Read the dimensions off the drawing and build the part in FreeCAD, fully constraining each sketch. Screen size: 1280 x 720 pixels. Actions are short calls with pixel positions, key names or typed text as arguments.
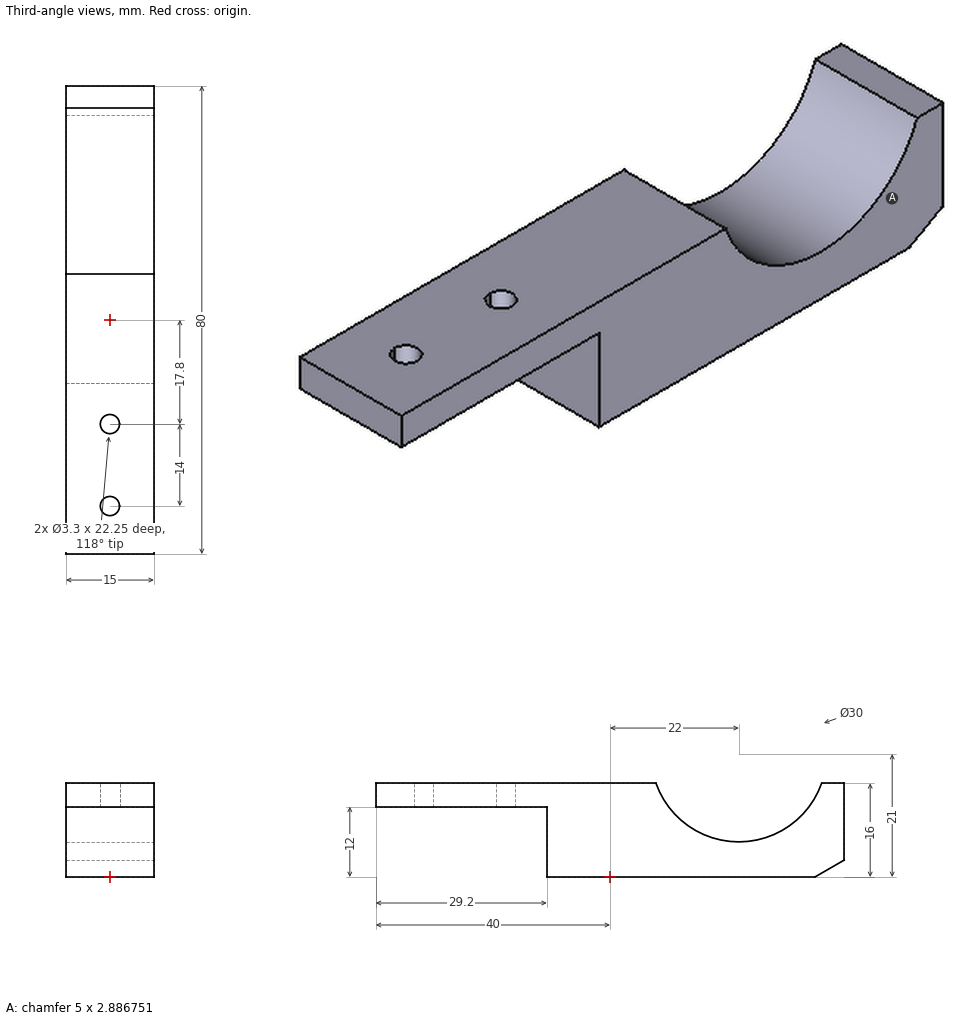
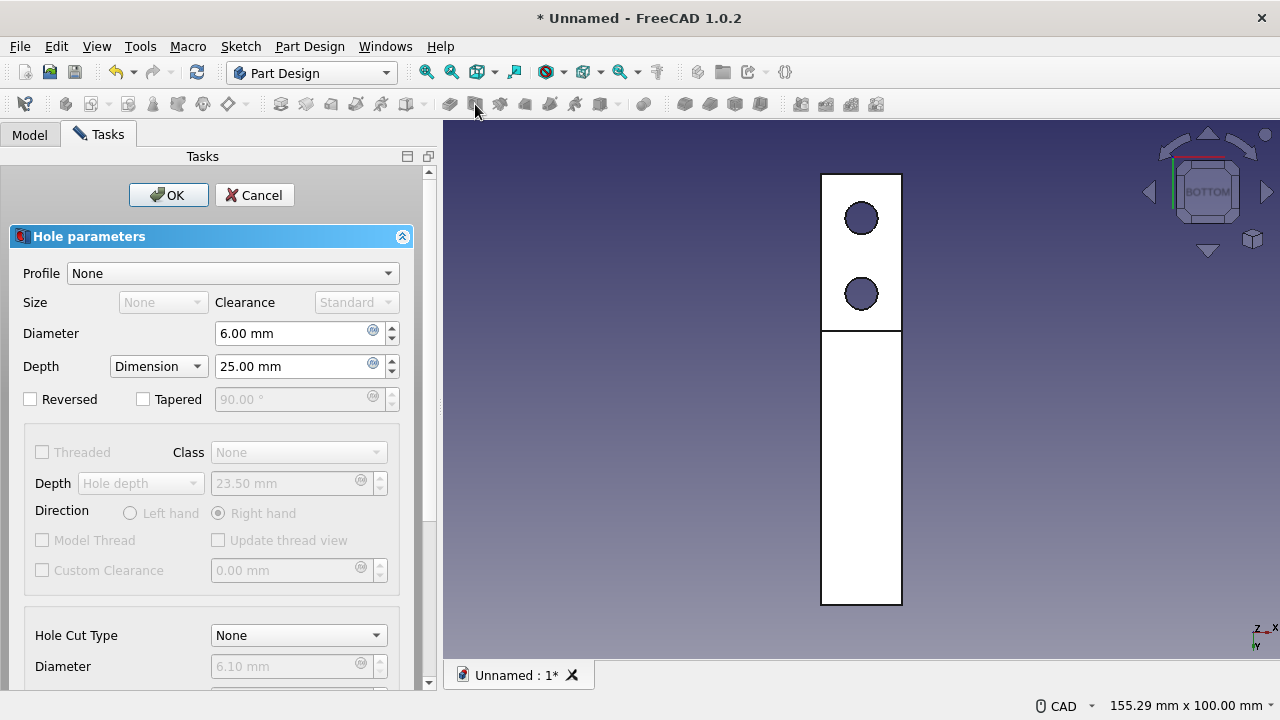
triple_click(300, 334)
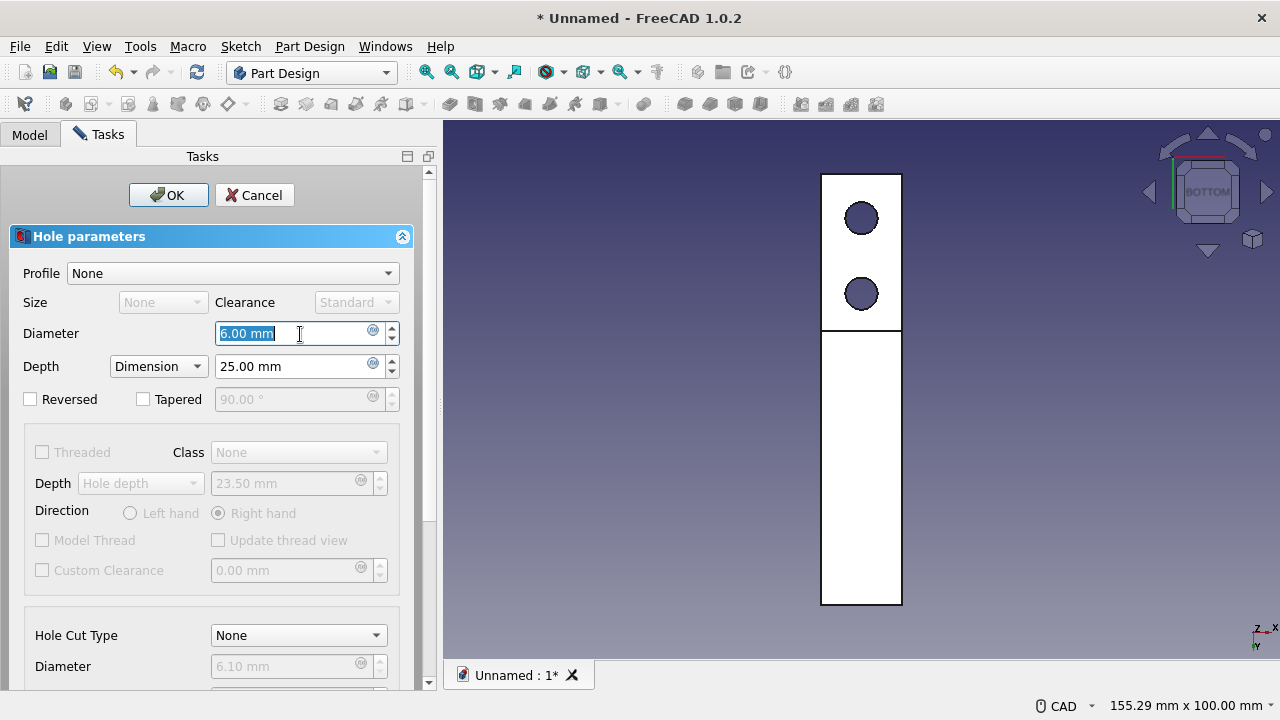
text(3.3)
key(Tab)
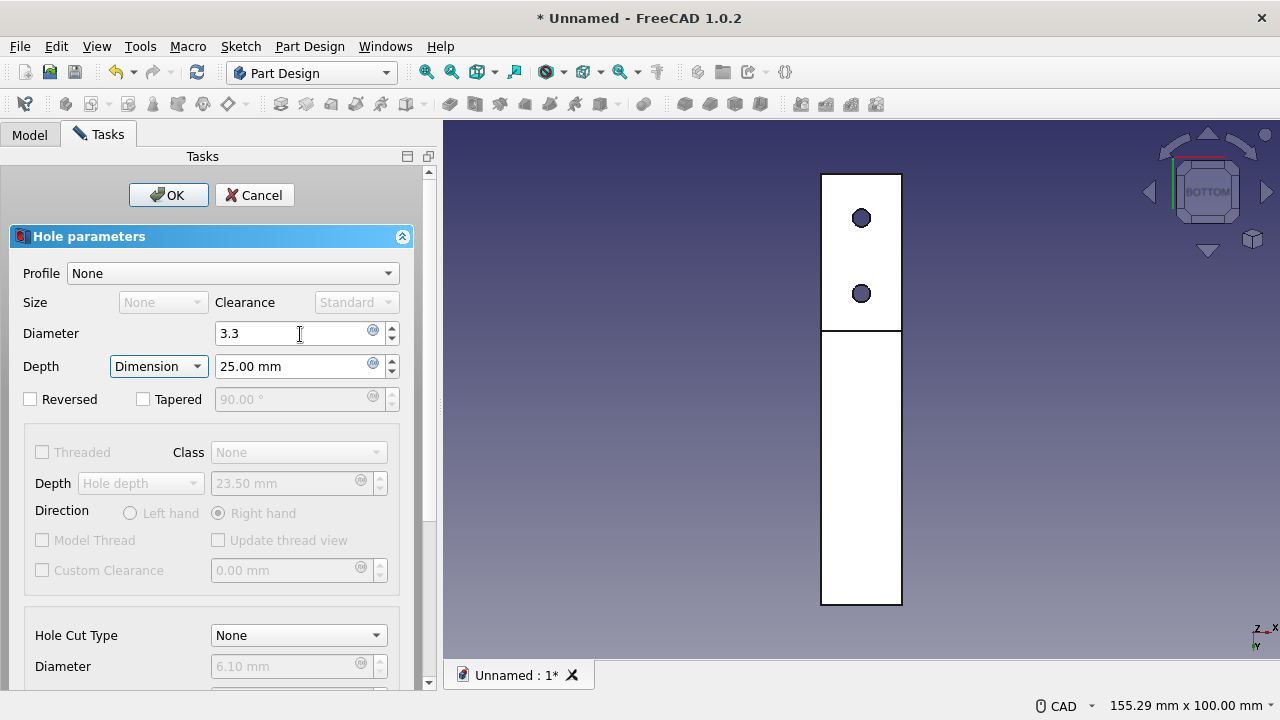
triple_click(300, 366)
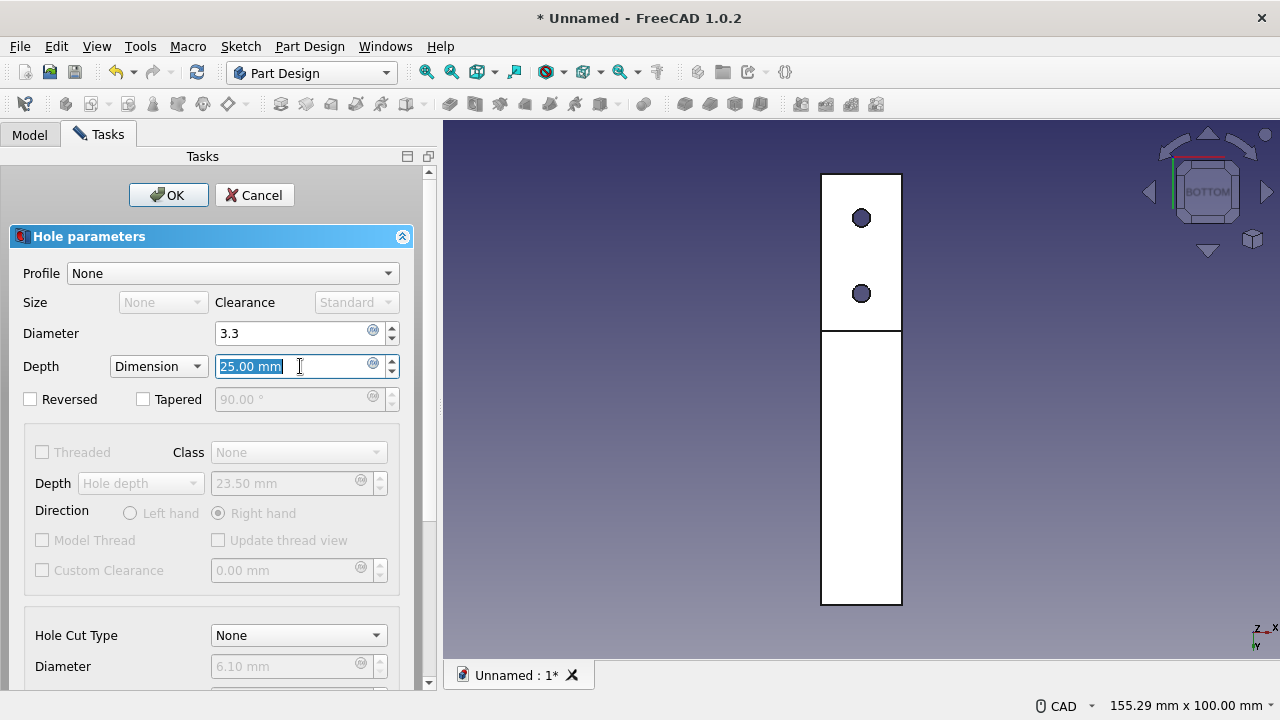
text(22.25)
key(Tab)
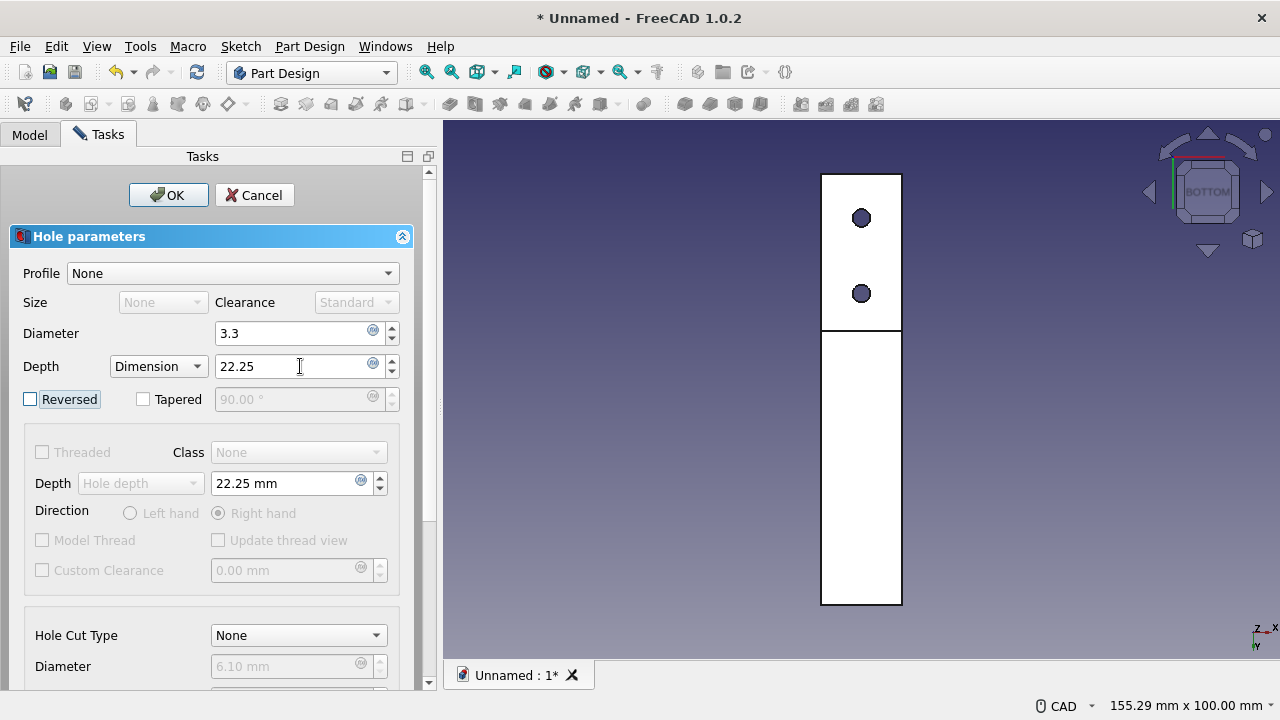
click(169, 195)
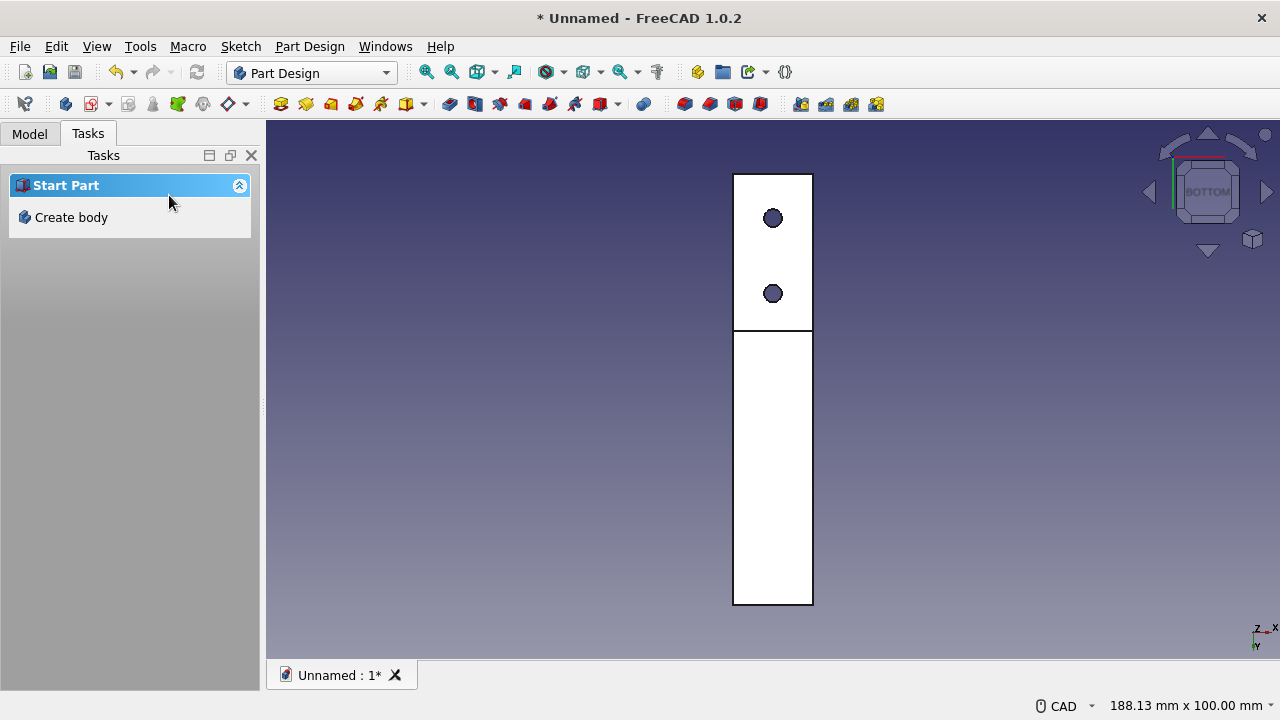
click(773, 604)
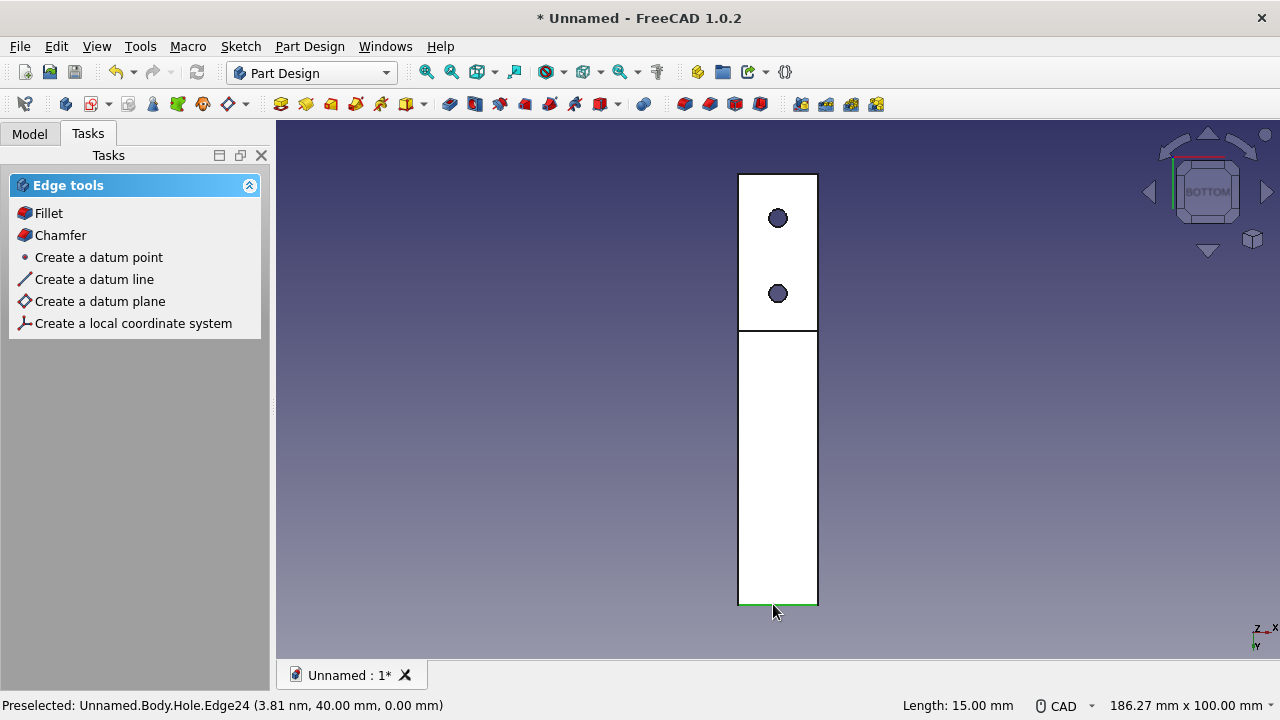
click(710, 104)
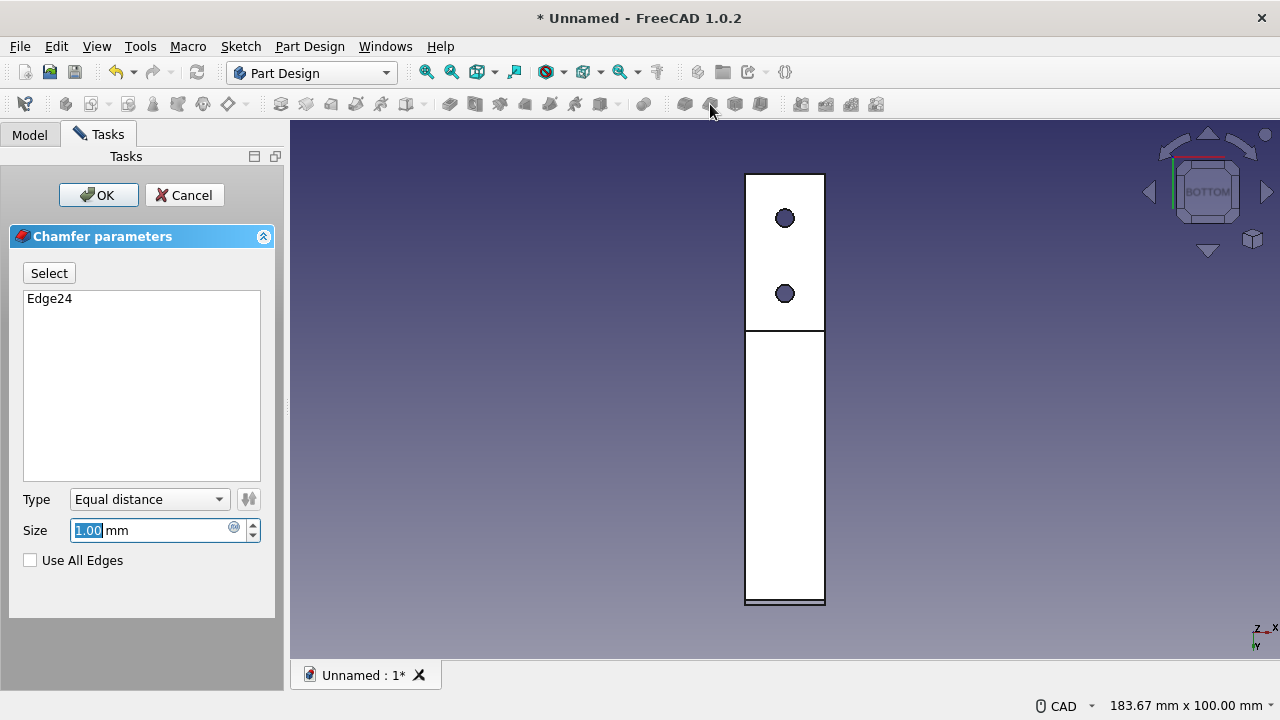
text(5)
key(Tab)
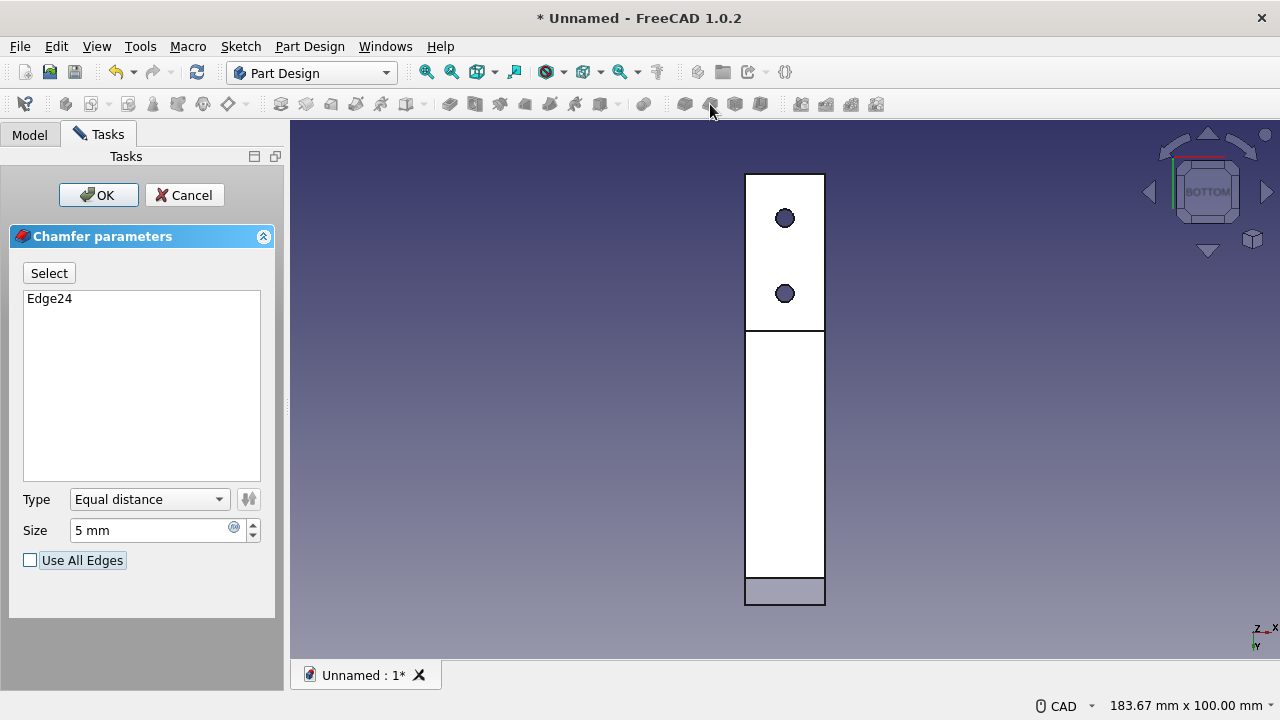
click(150, 500)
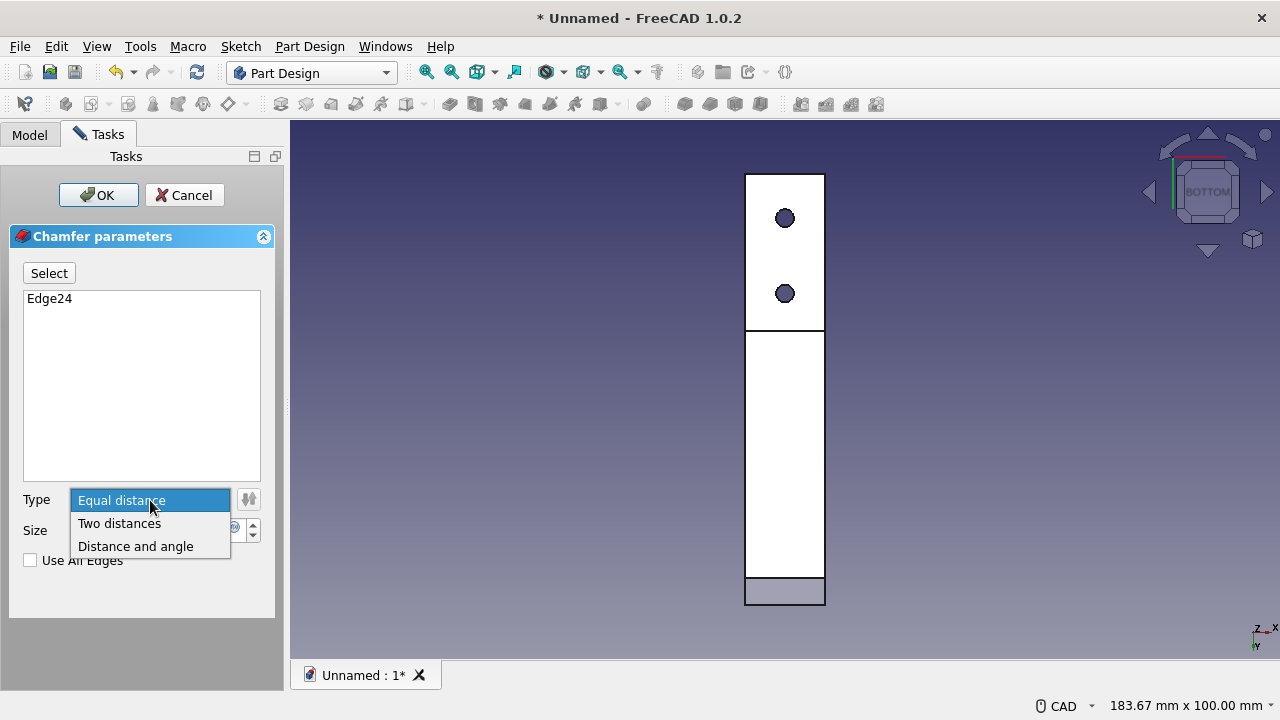
click(148, 524)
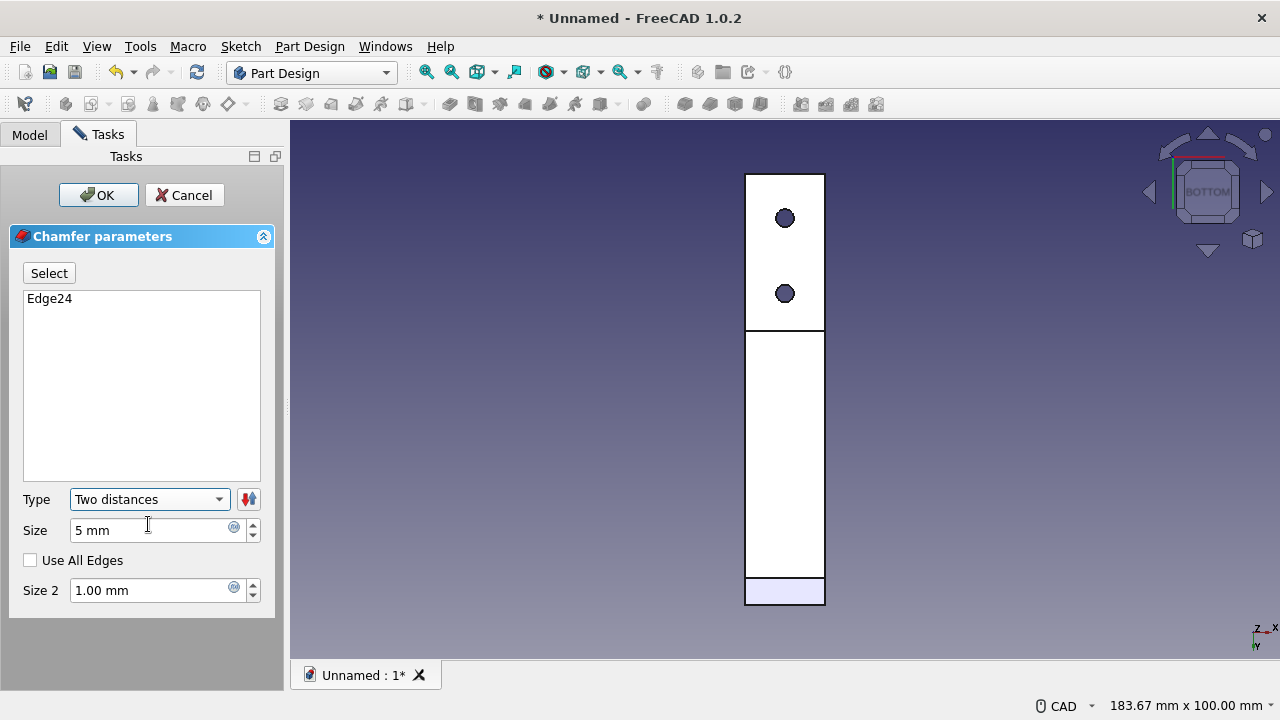
triple_click(158, 590)